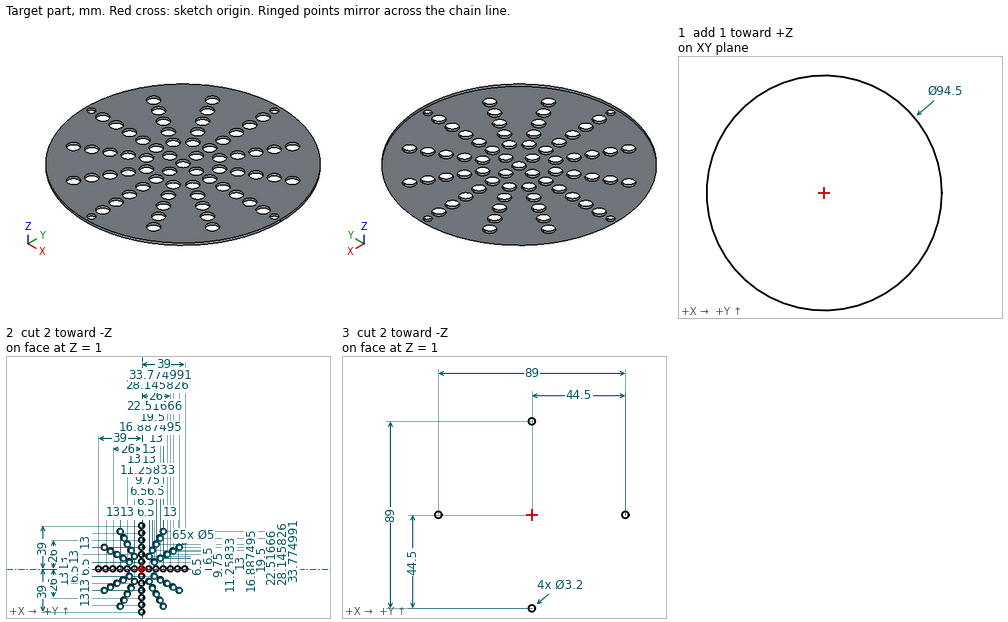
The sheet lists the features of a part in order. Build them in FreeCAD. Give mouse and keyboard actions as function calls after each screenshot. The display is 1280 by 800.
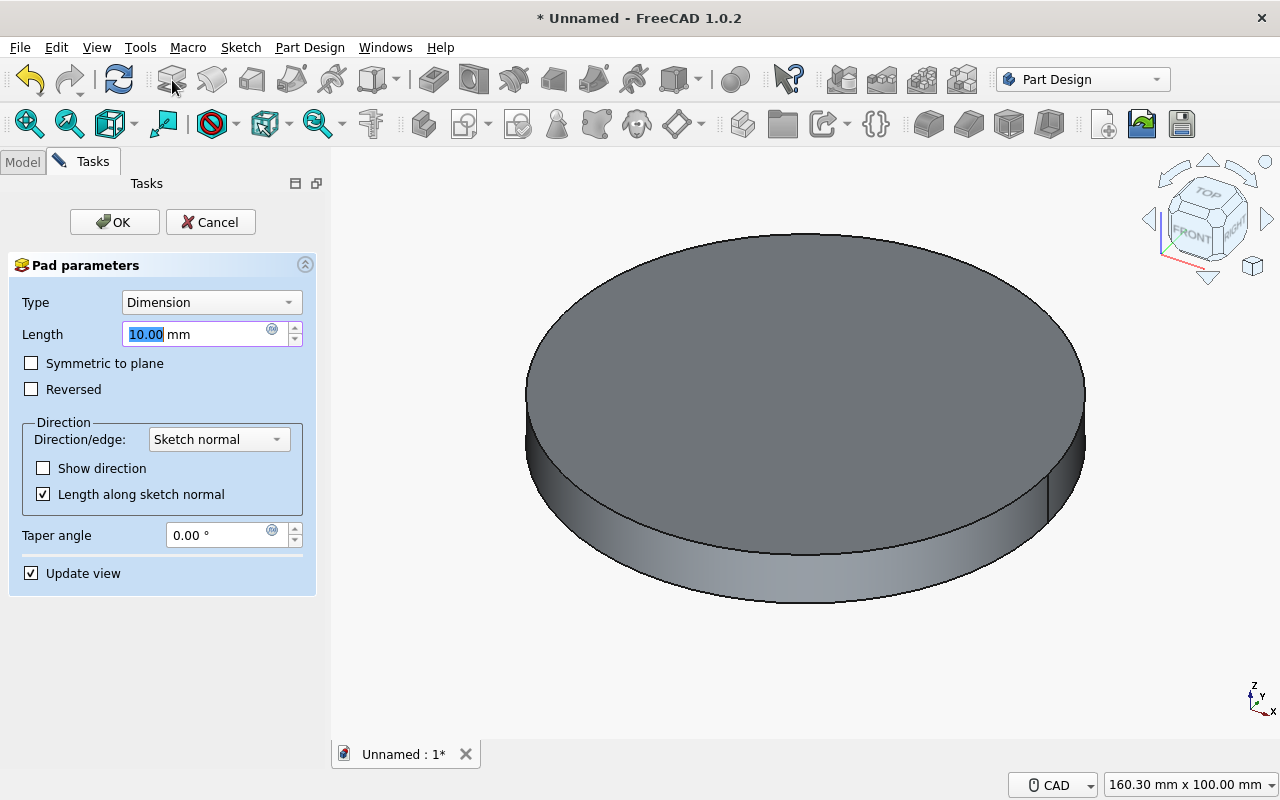
text(1)
key(Tab)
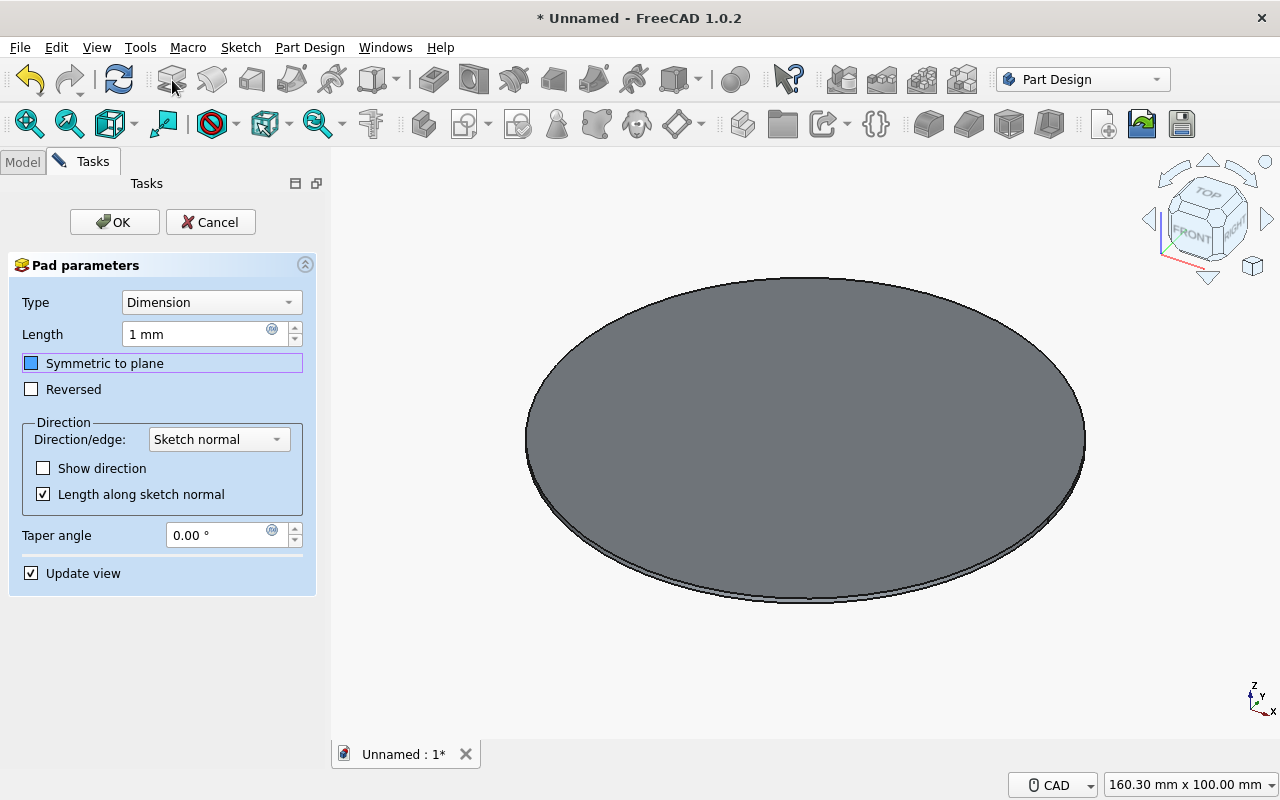
click(115, 222)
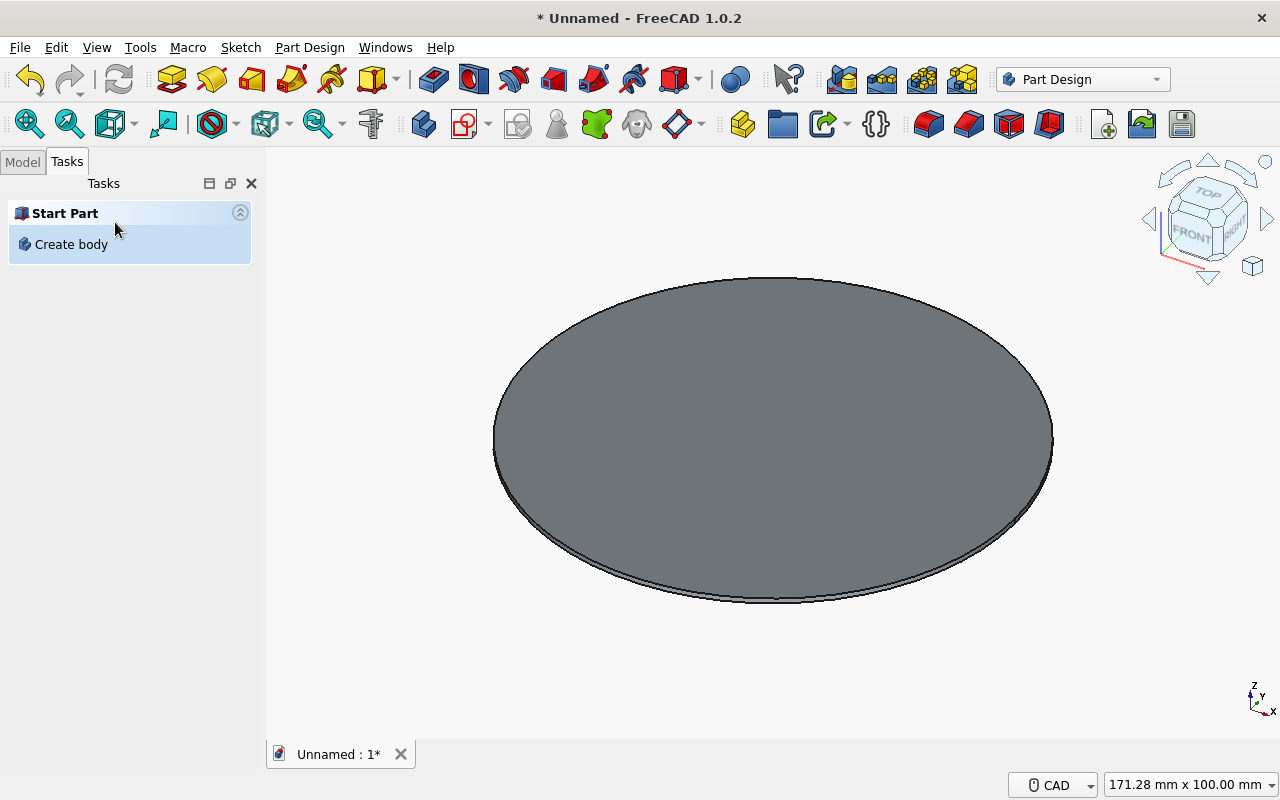
click(773, 437)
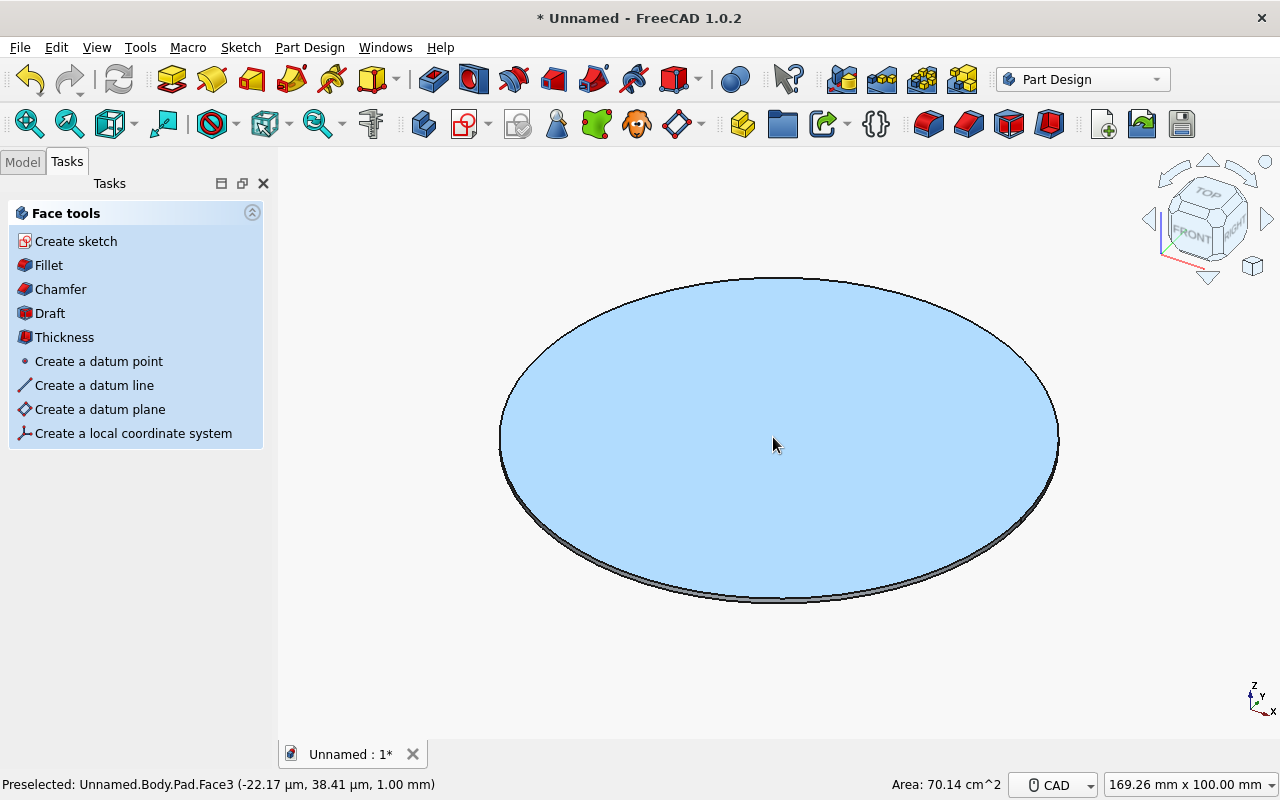
click(464, 124)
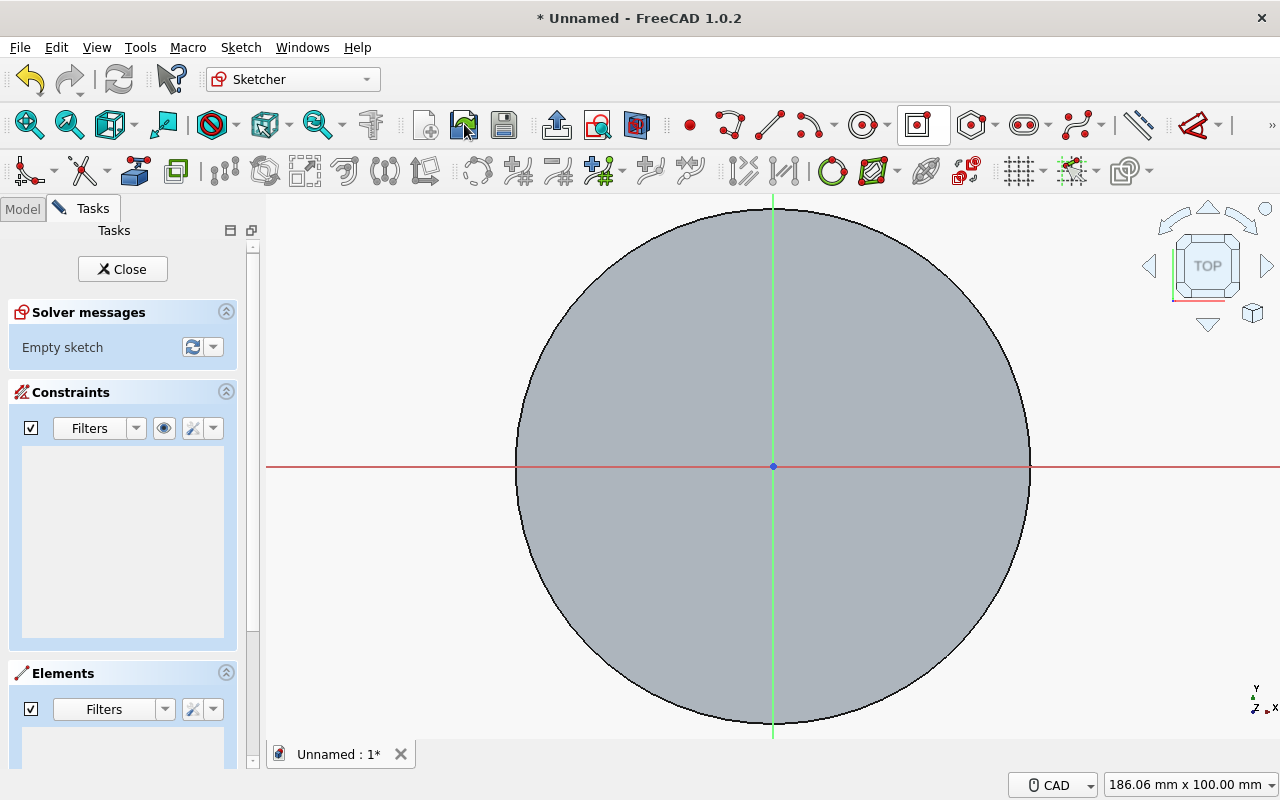
scroll(395, 467, down, 1)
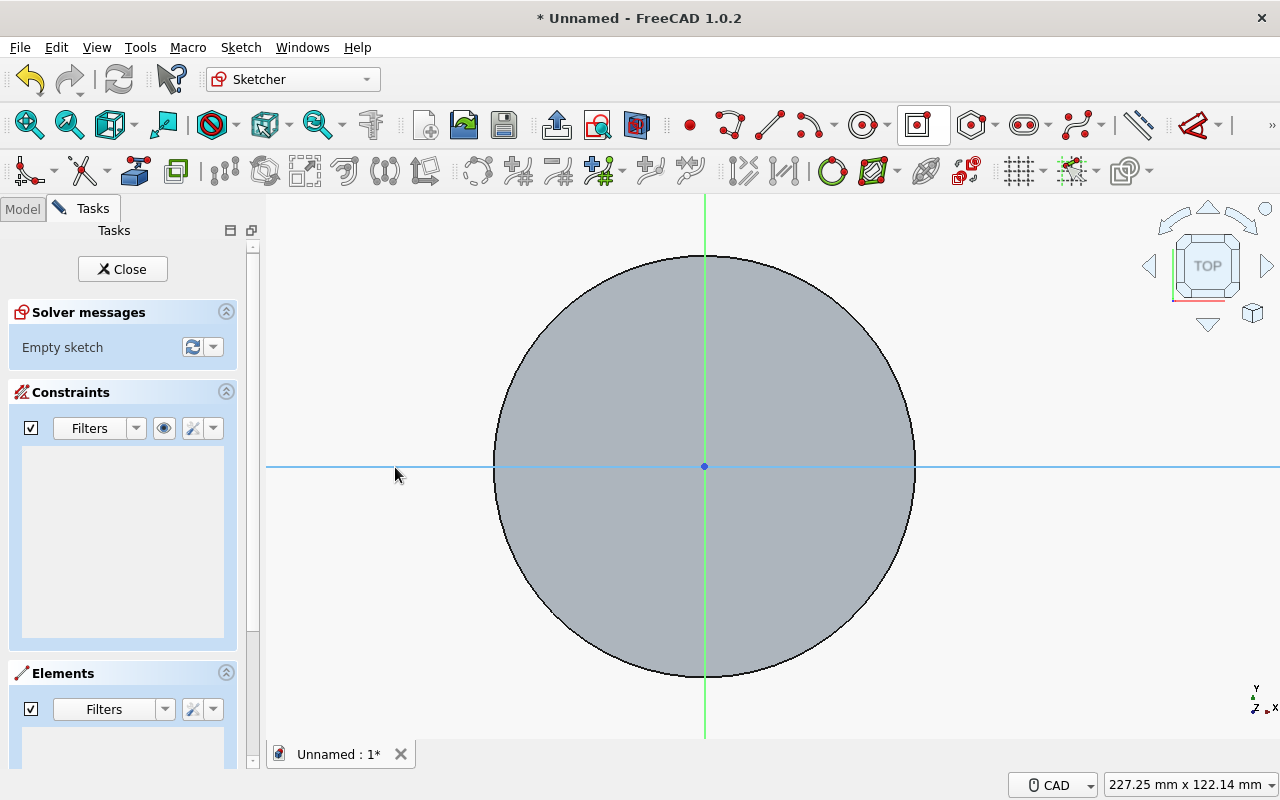
key(g)
key(c)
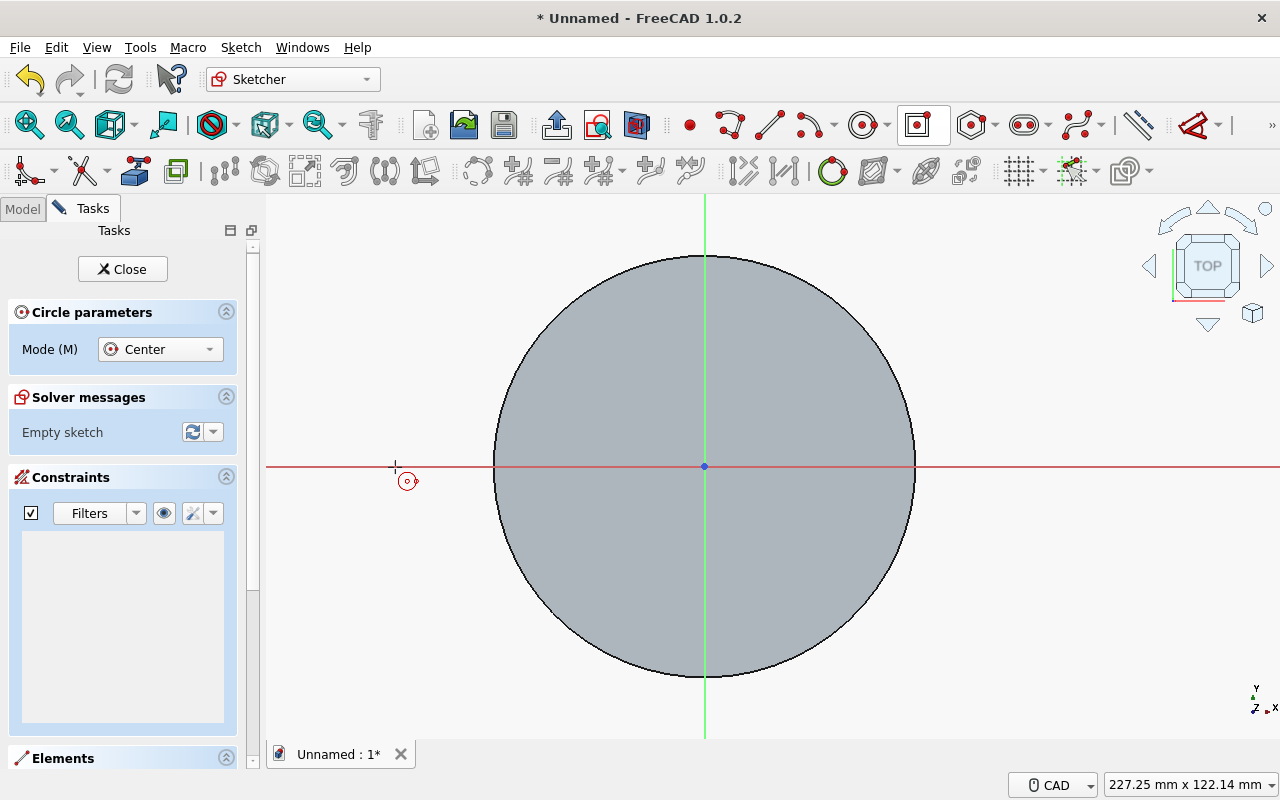
scroll(705, 438, up, 4)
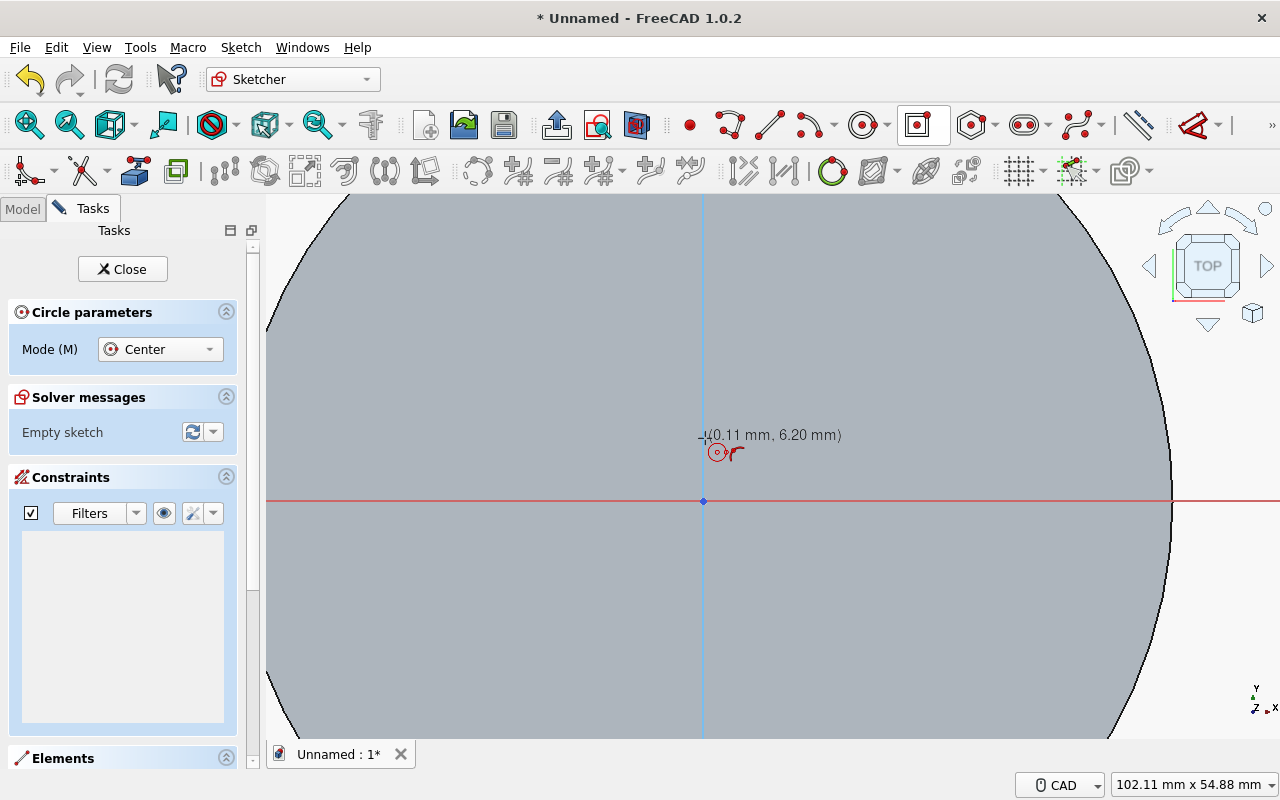
click(703, 437)
move(721, 419)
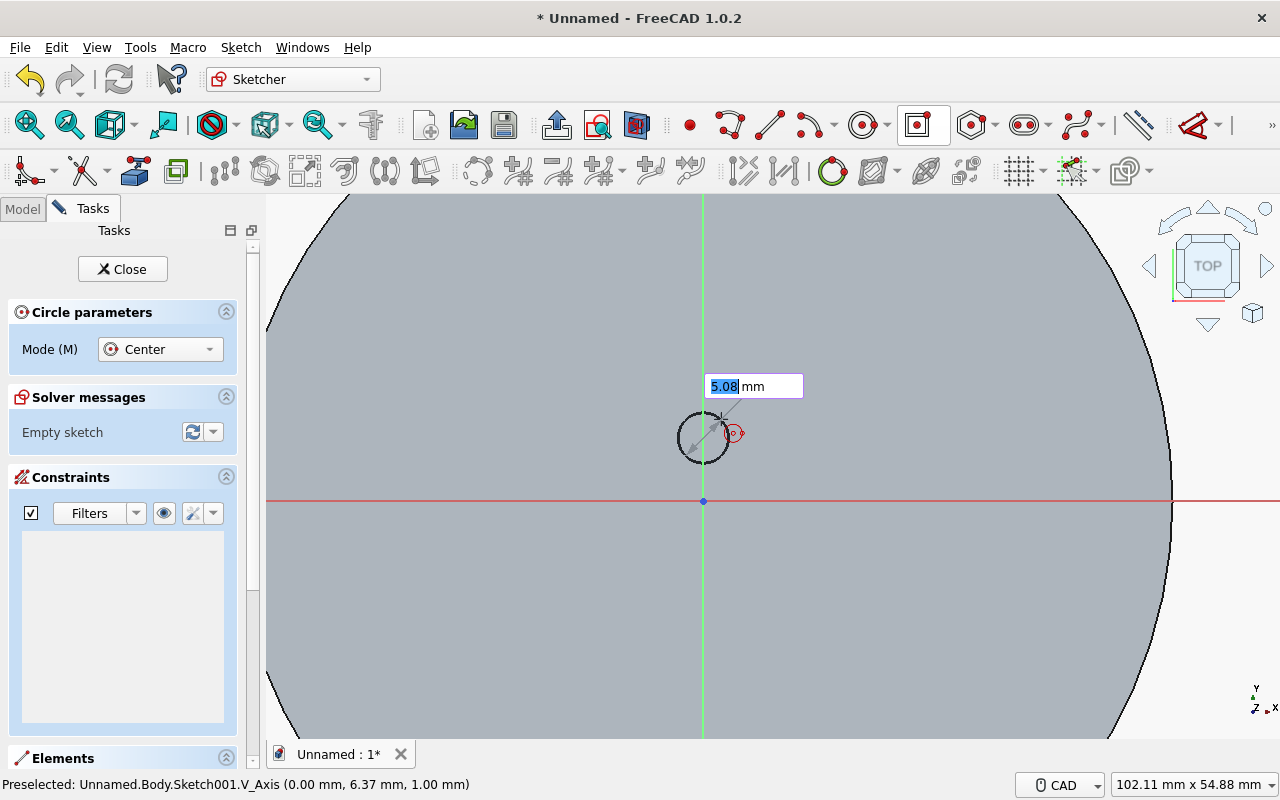
text(5)
key(Return)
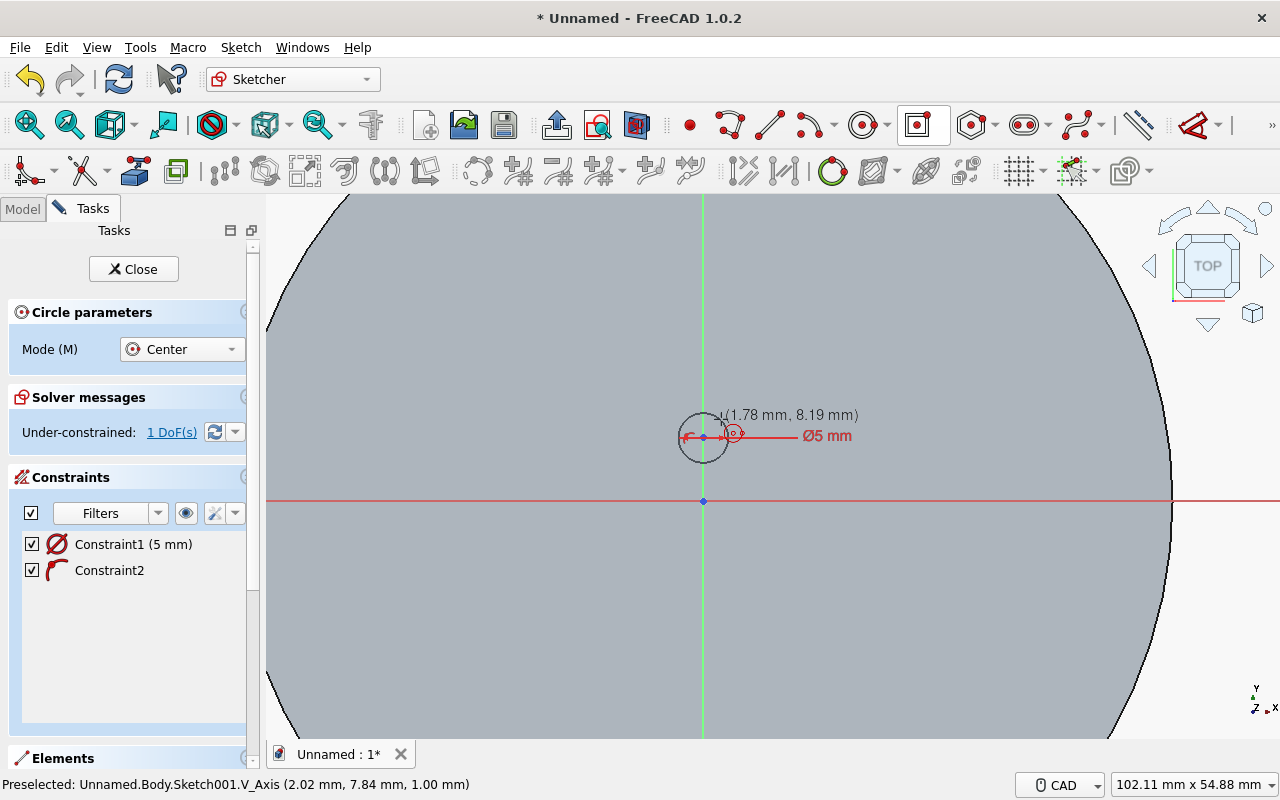
click(703, 372)
move(721, 355)